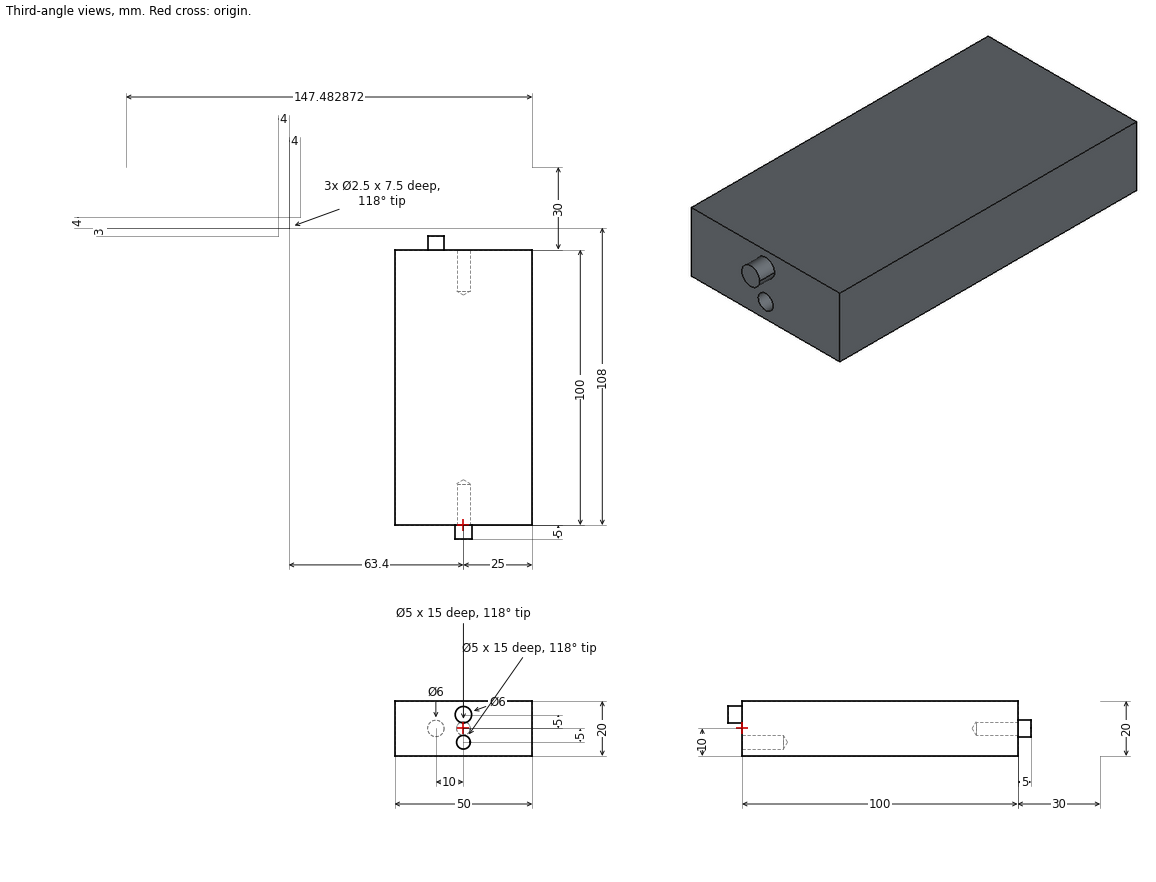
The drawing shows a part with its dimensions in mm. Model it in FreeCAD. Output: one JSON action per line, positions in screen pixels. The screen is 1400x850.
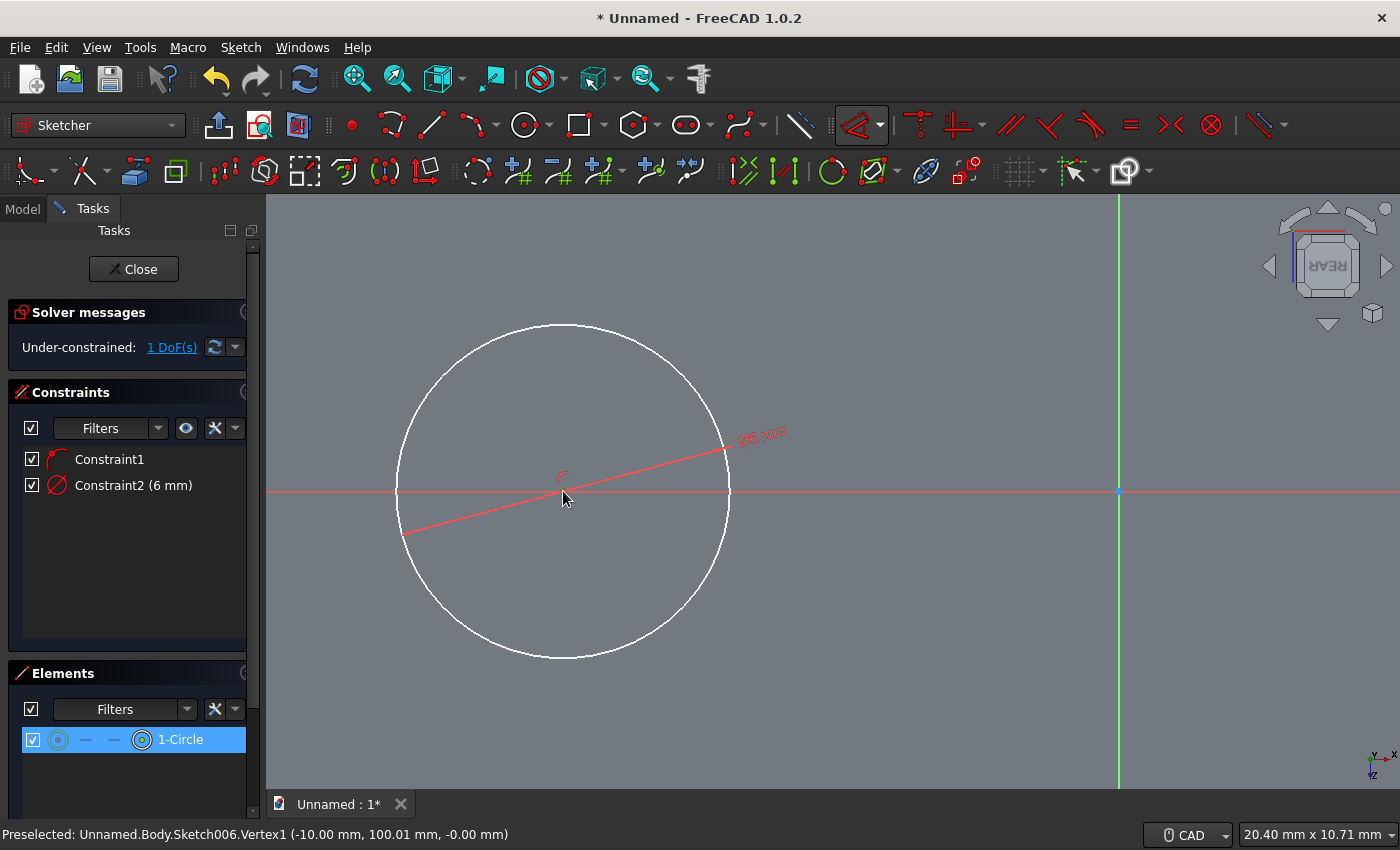
{"action": "key", "text": "l"}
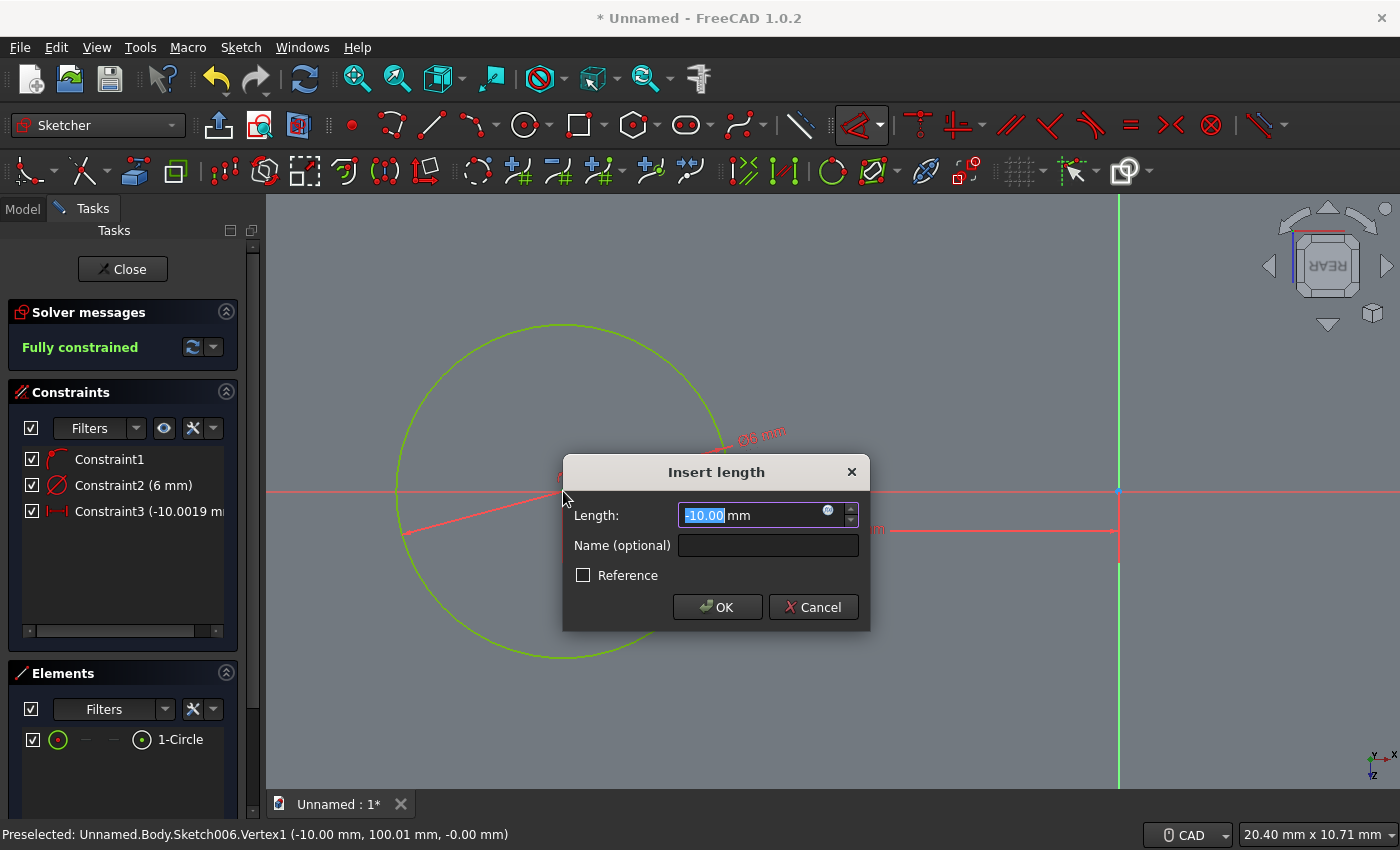
{"action": "type", "text": "-10"}
{"action": "key", "text": "Return"}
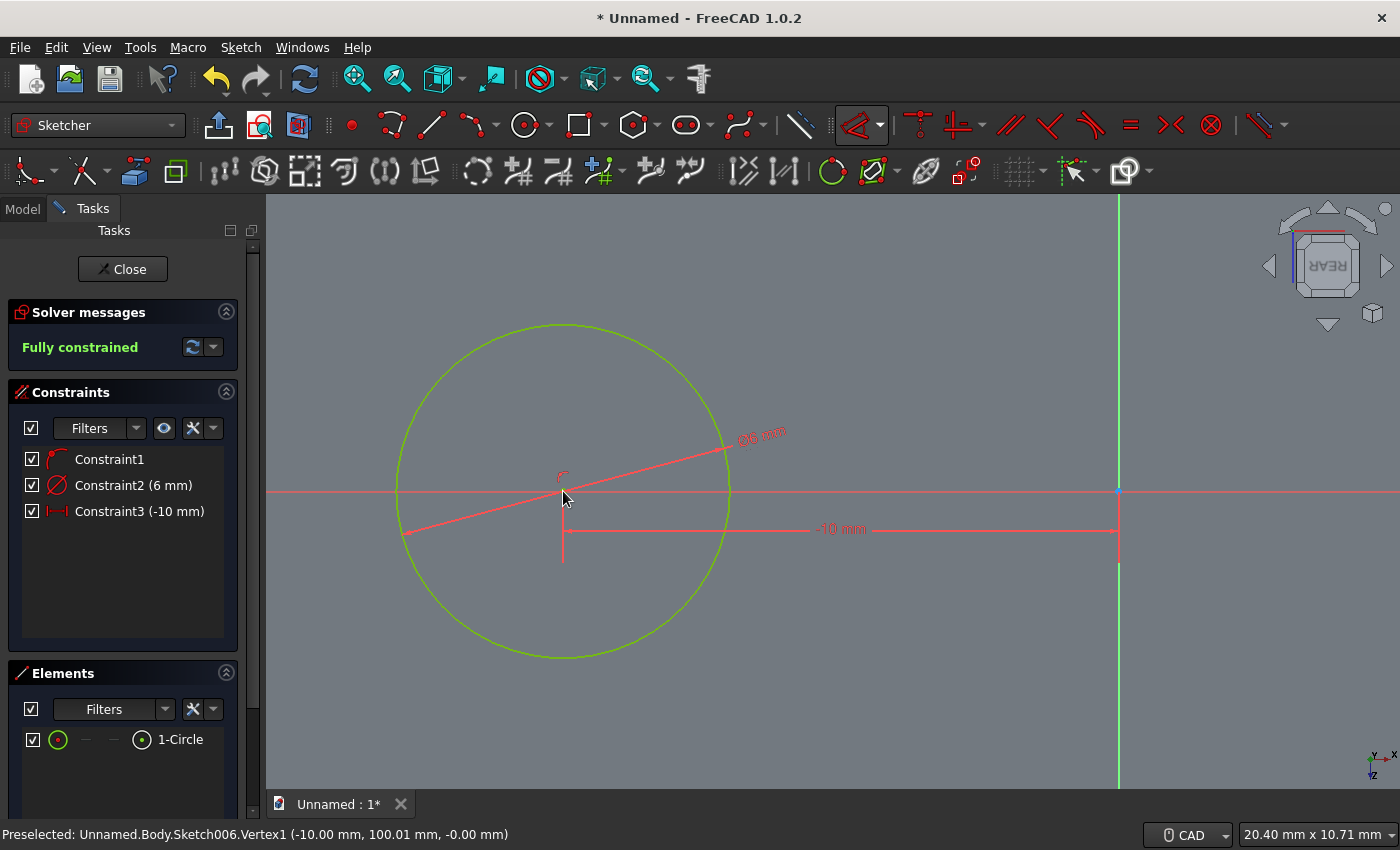
{"action": "left_click", "coordinate": [123, 269]}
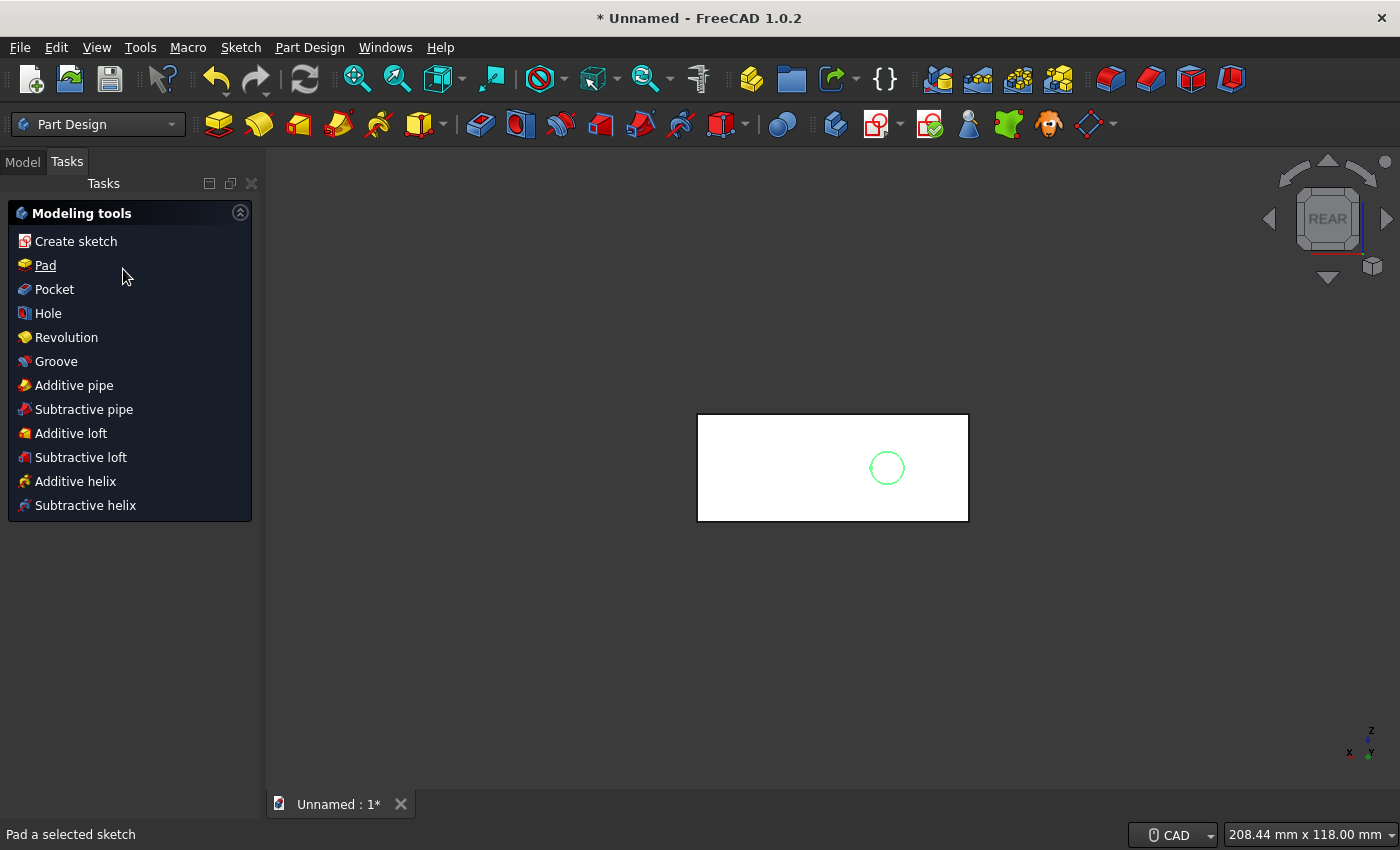
{"action": "left_click", "coordinate": [220, 124]}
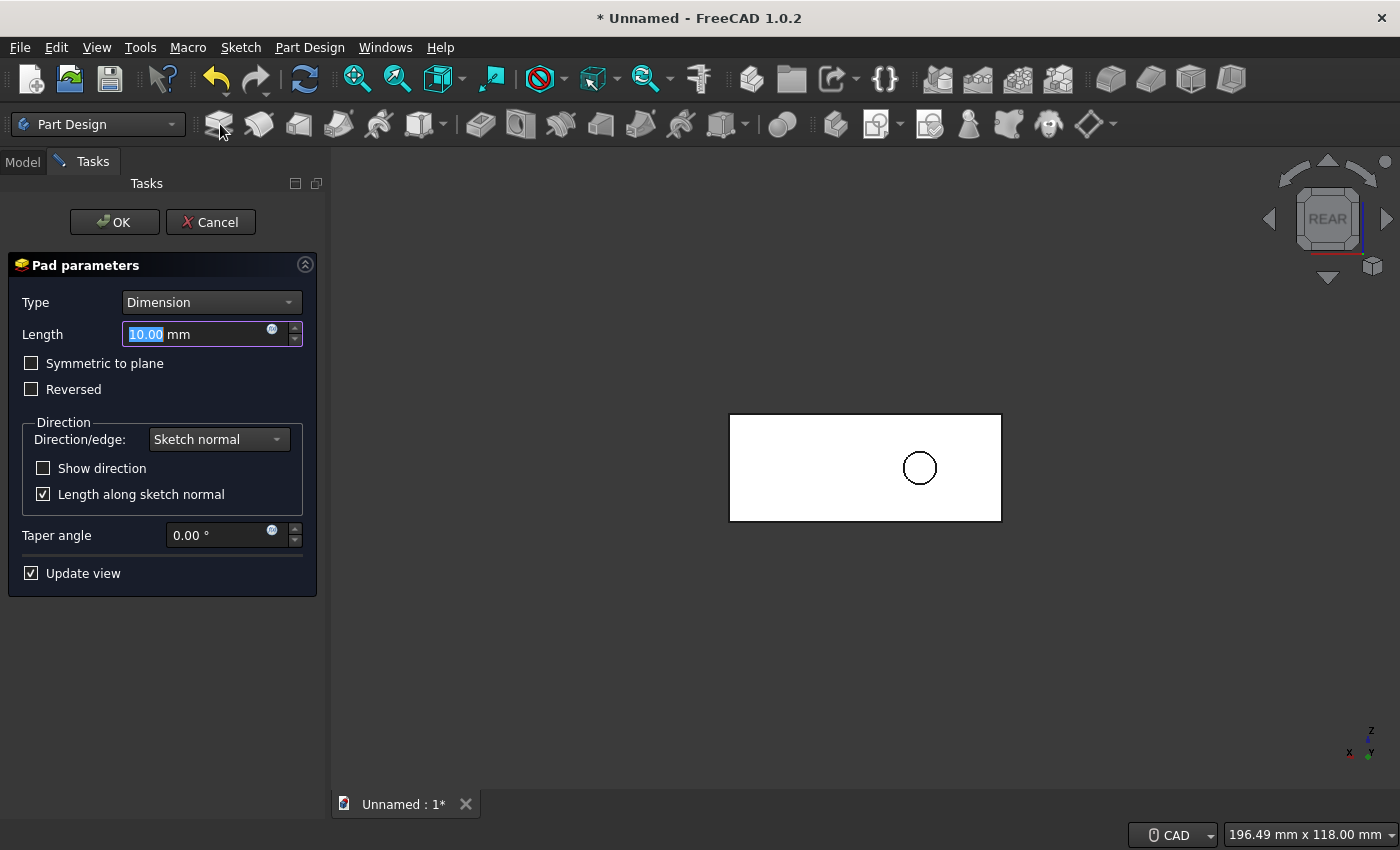
{"action": "type", "text": "5"}
{"action": "key", "text": "Tab"}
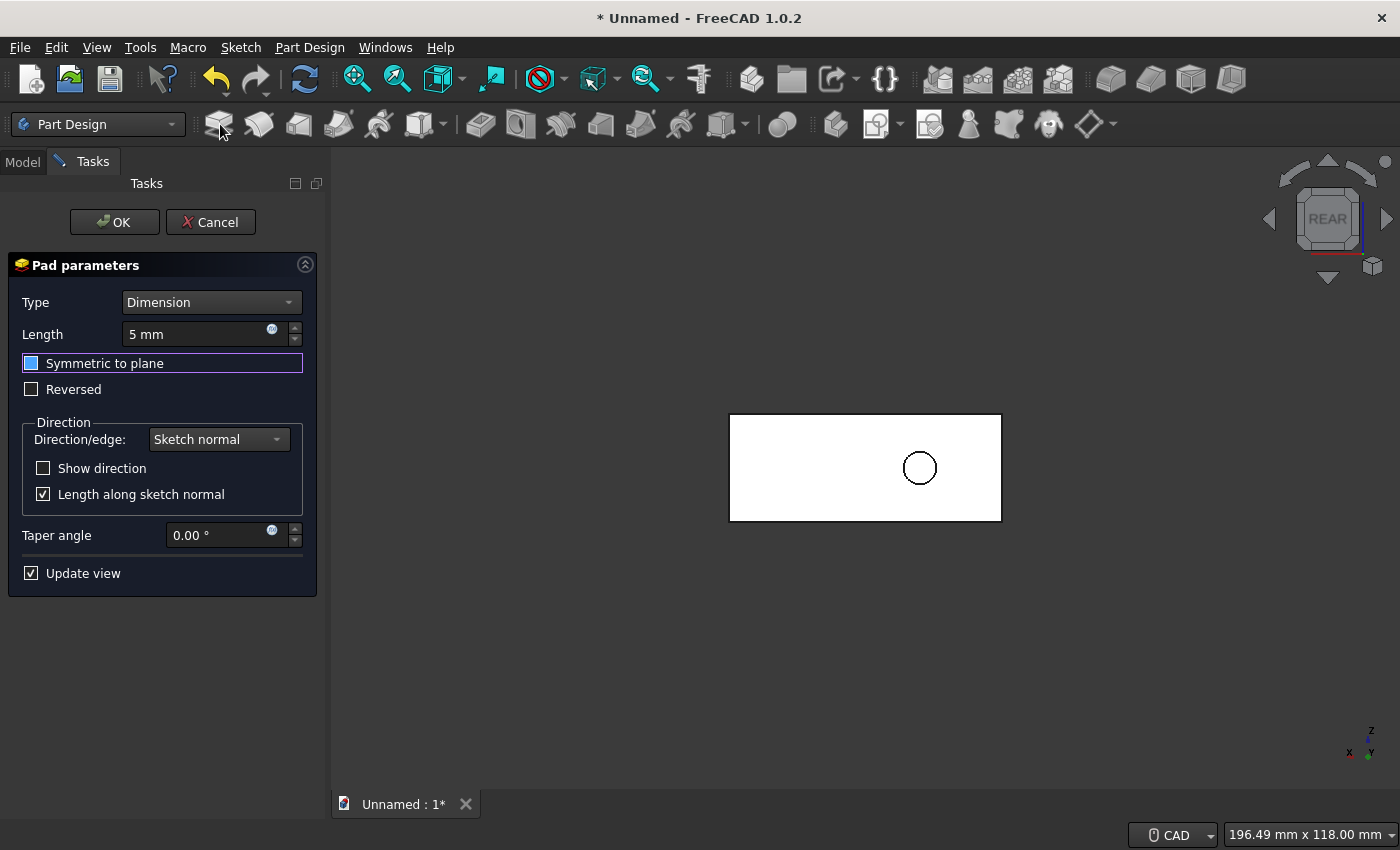
{"action": "left_click", "coordinate": [115, 222]}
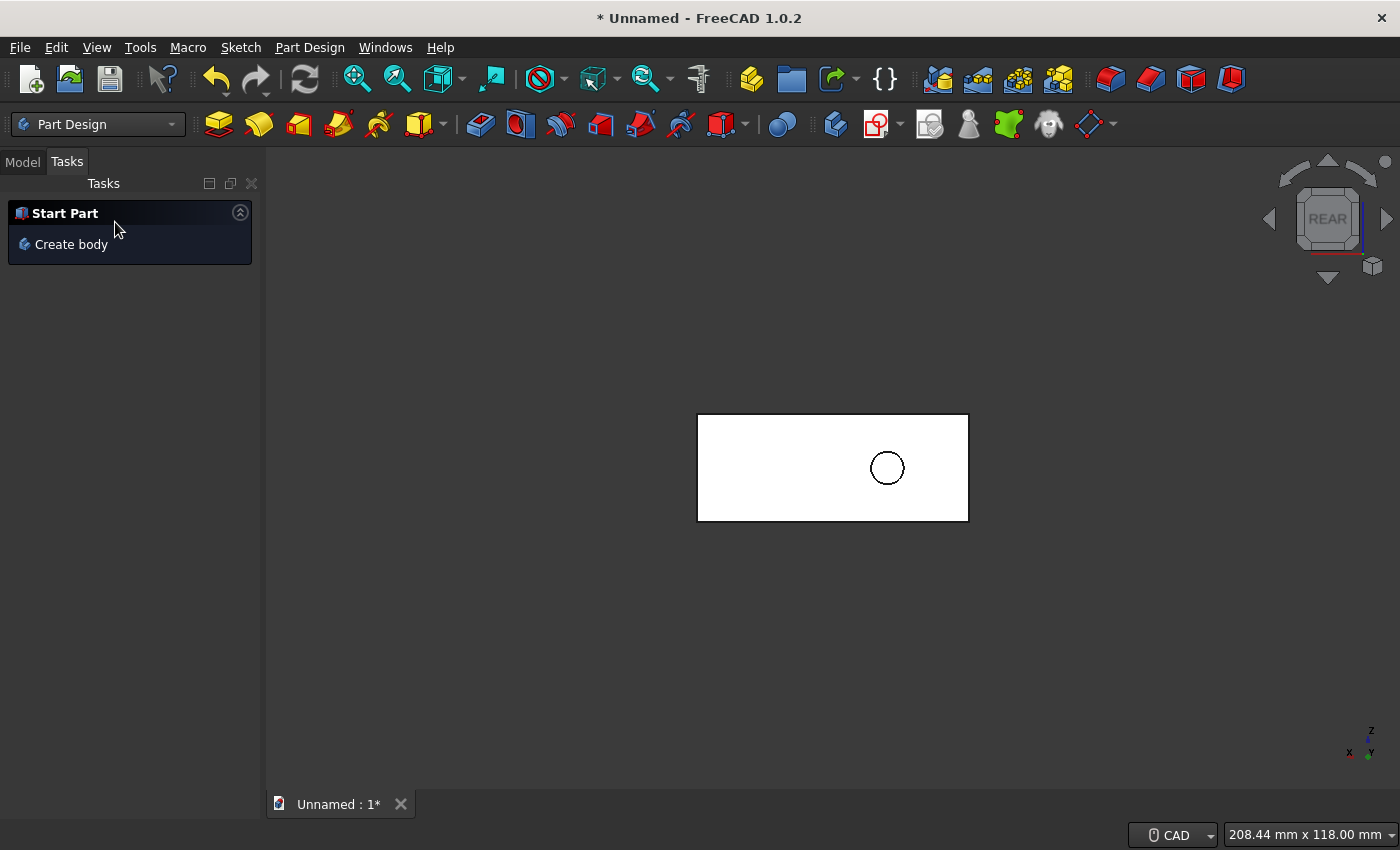
{"action": "key", "text": "v f"}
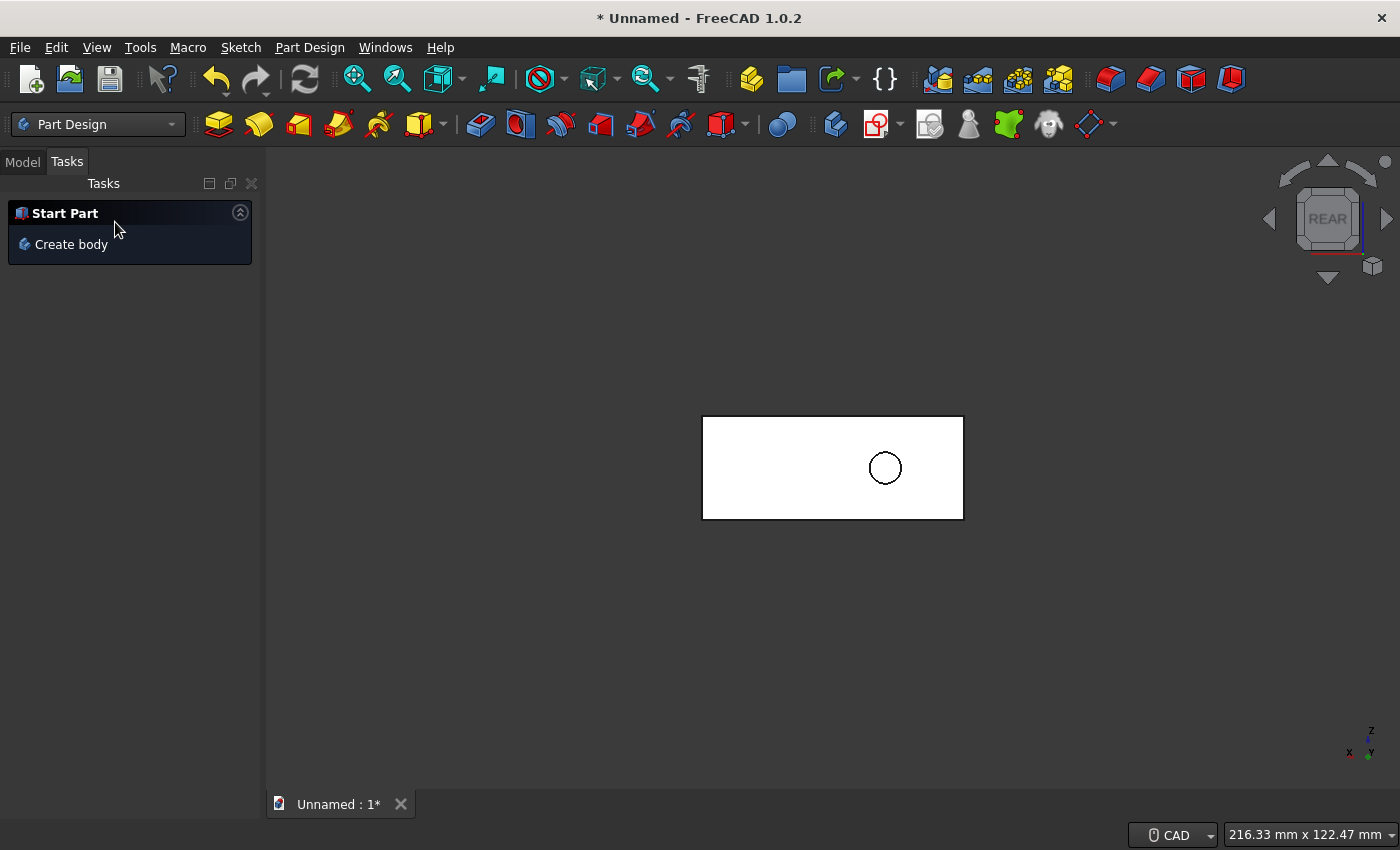
{"action": "left_click", "coordinate": [758, 467]}